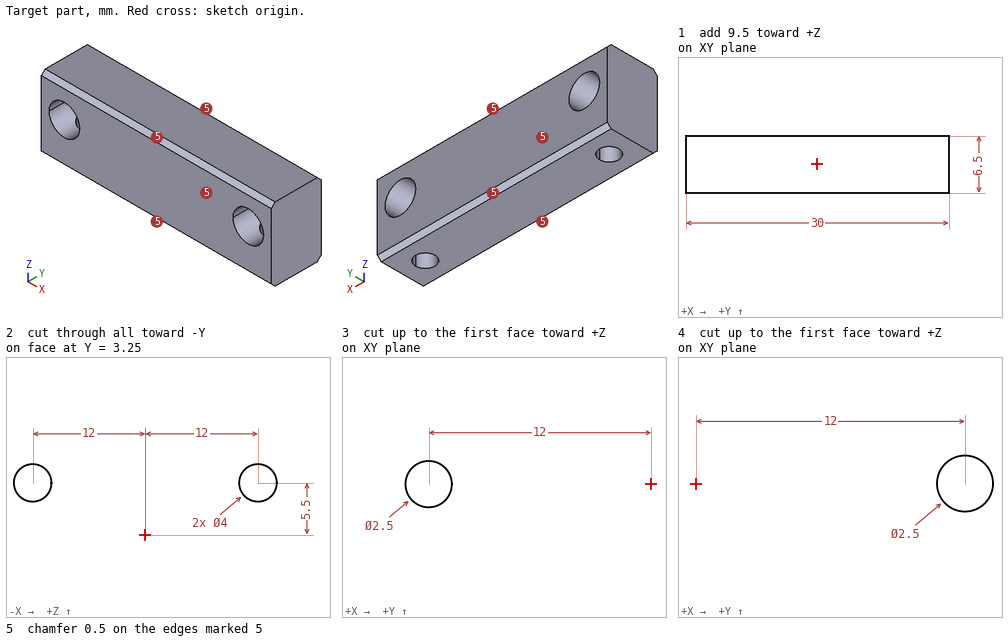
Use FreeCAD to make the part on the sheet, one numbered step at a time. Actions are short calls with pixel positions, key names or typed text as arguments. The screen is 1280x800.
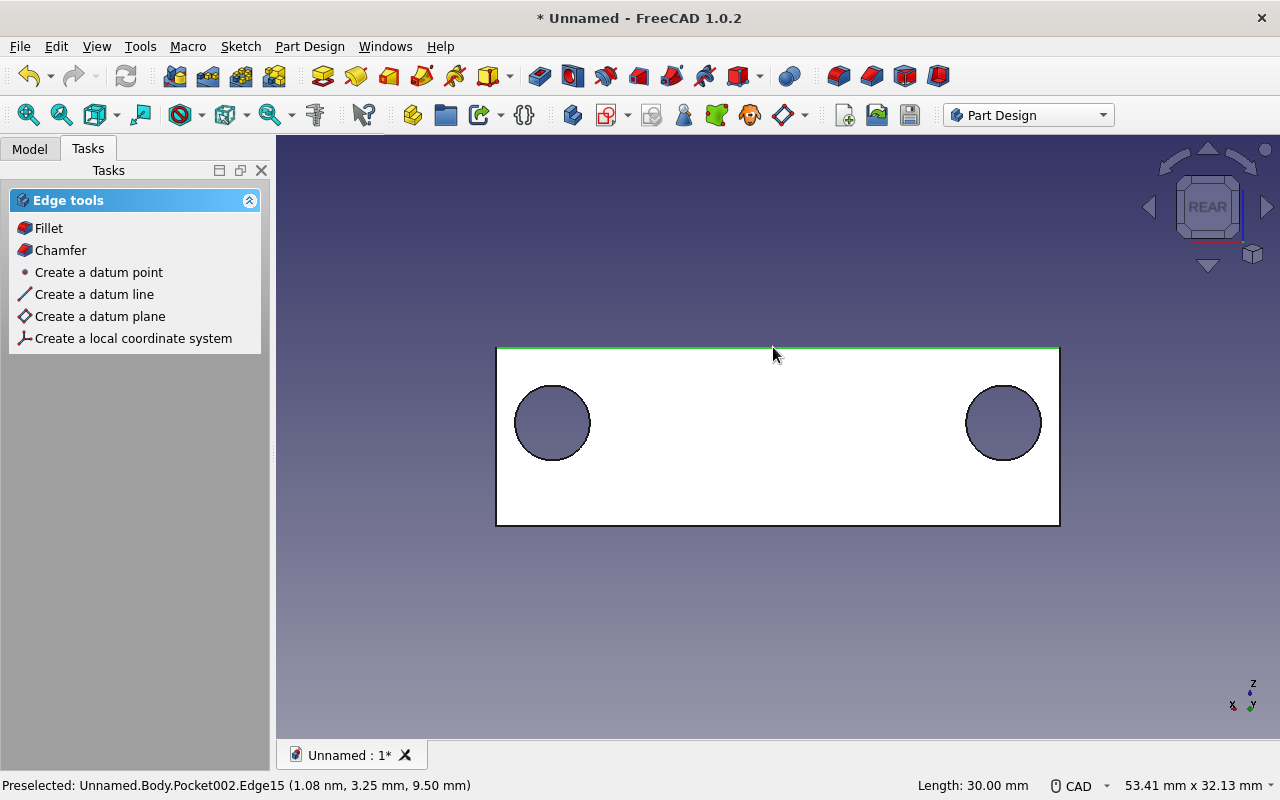
click(778, 525, ctrl)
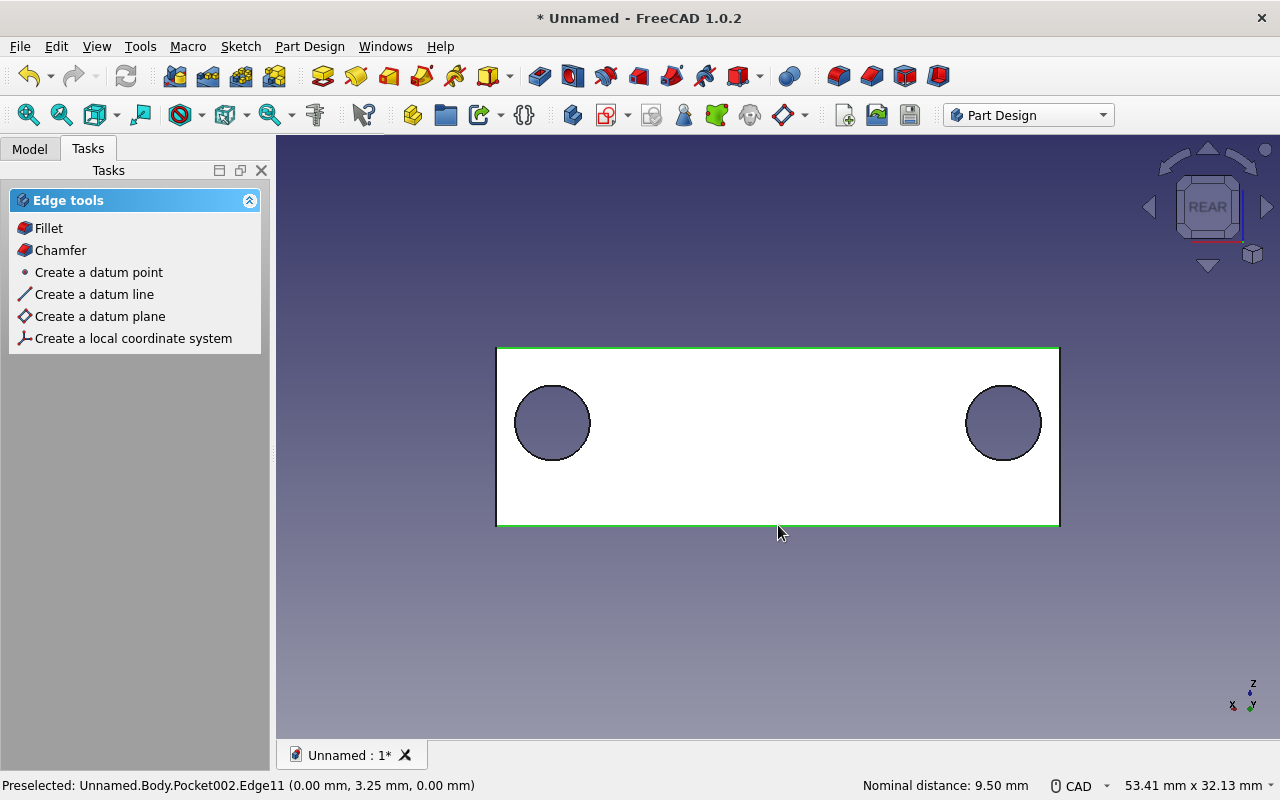
key(0)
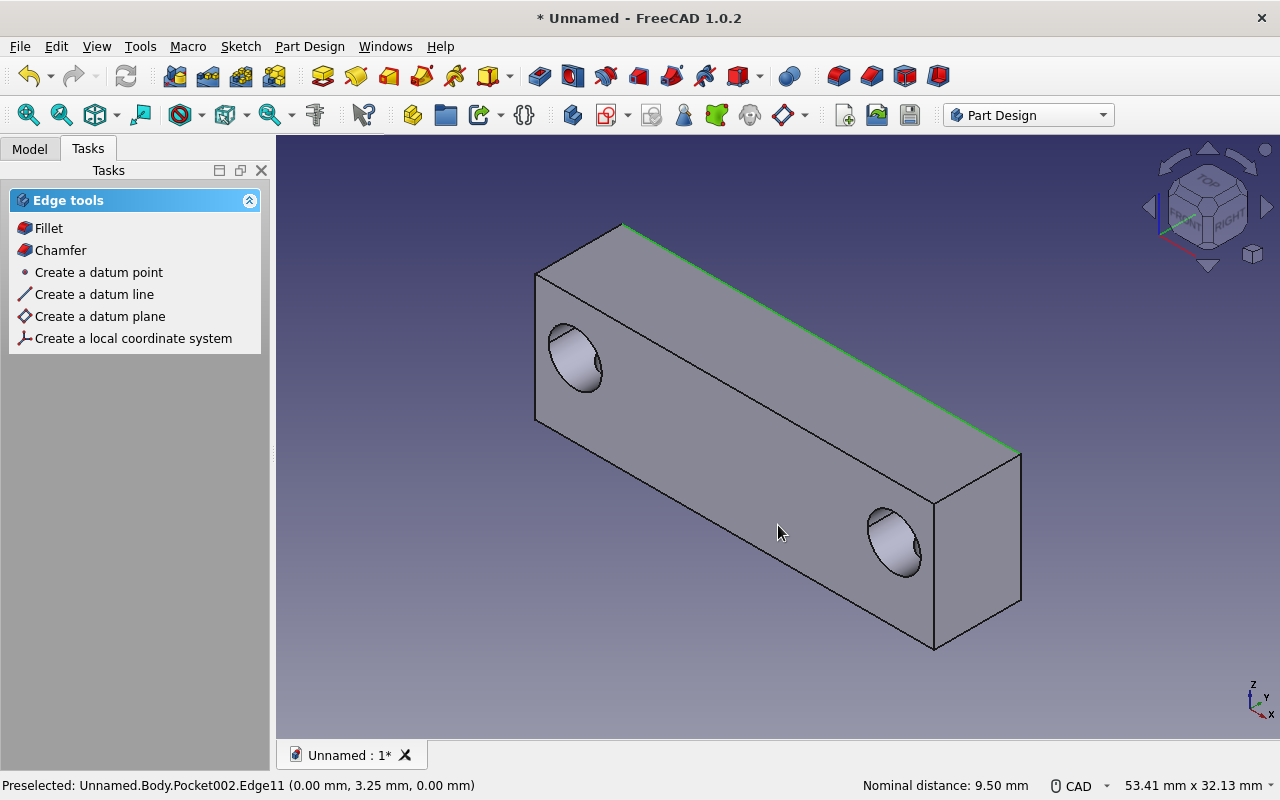
click(735, 388, ctrl)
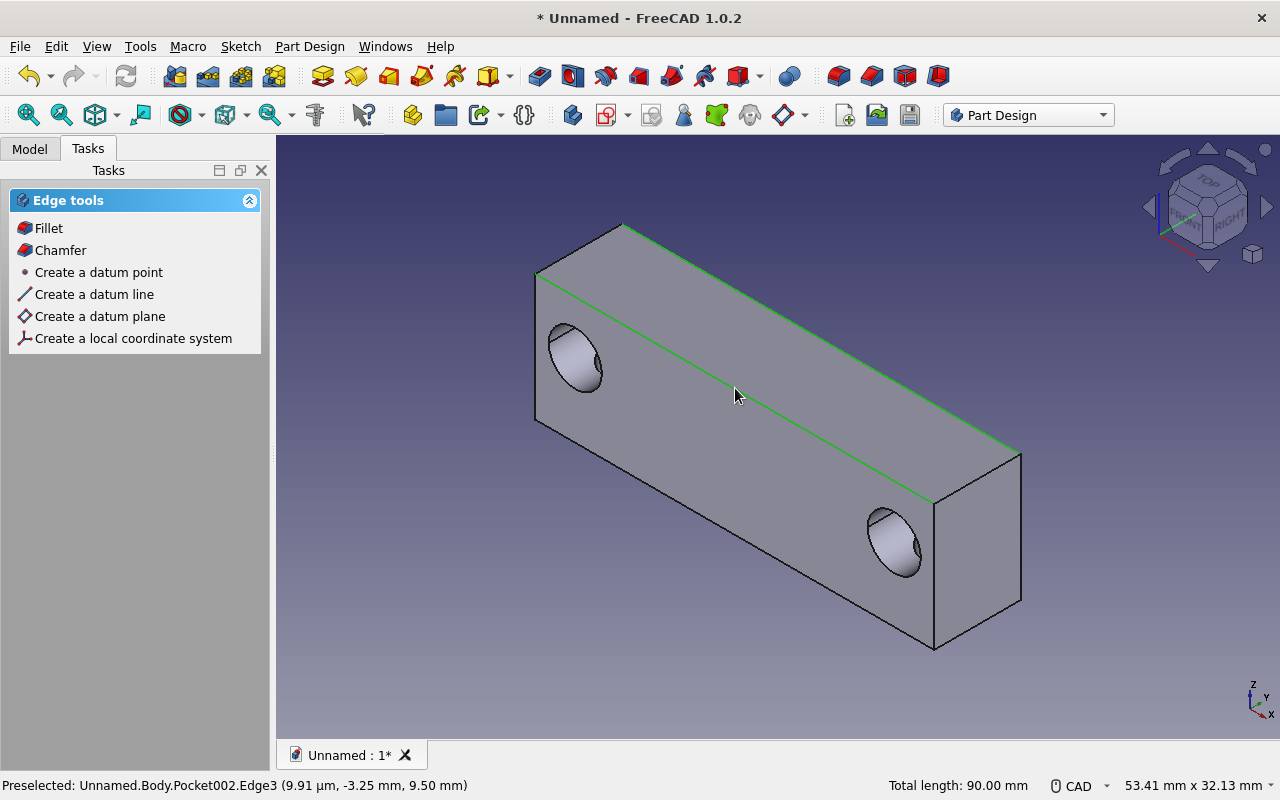
key(2)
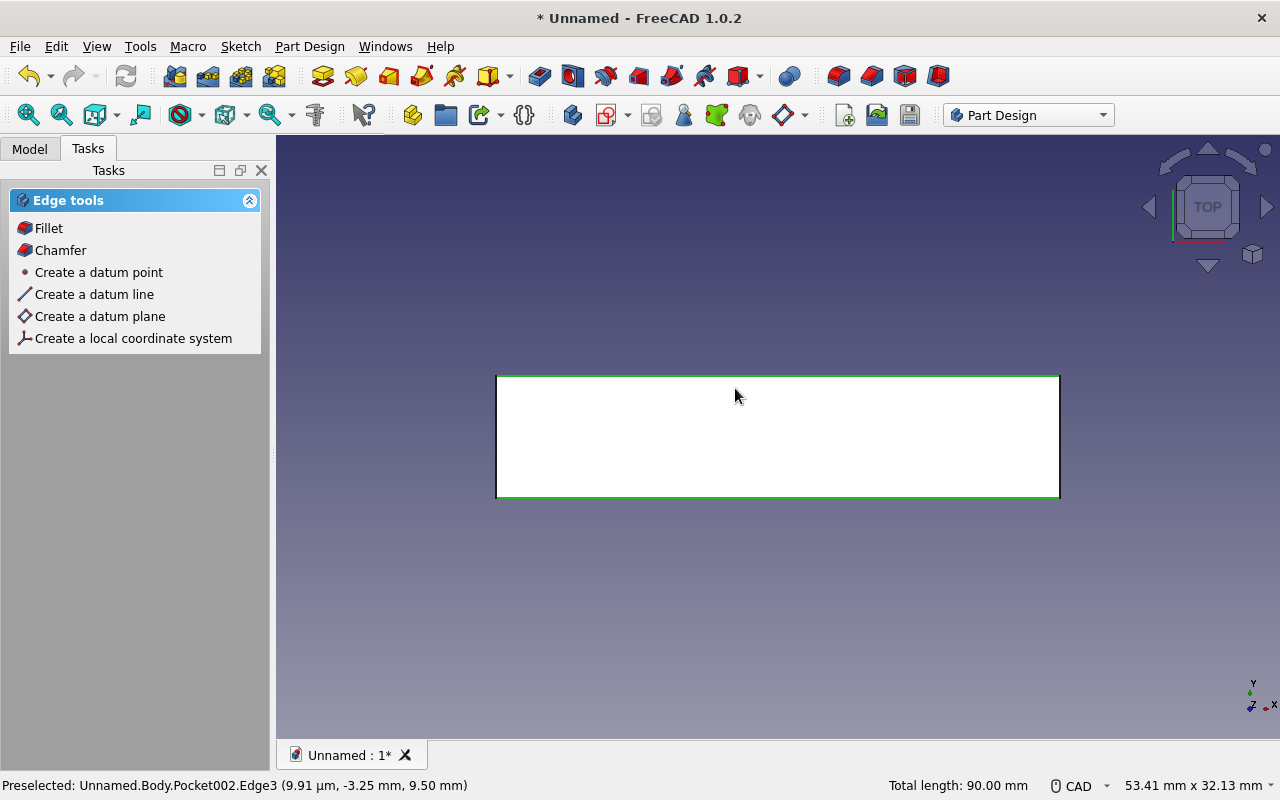
key(1)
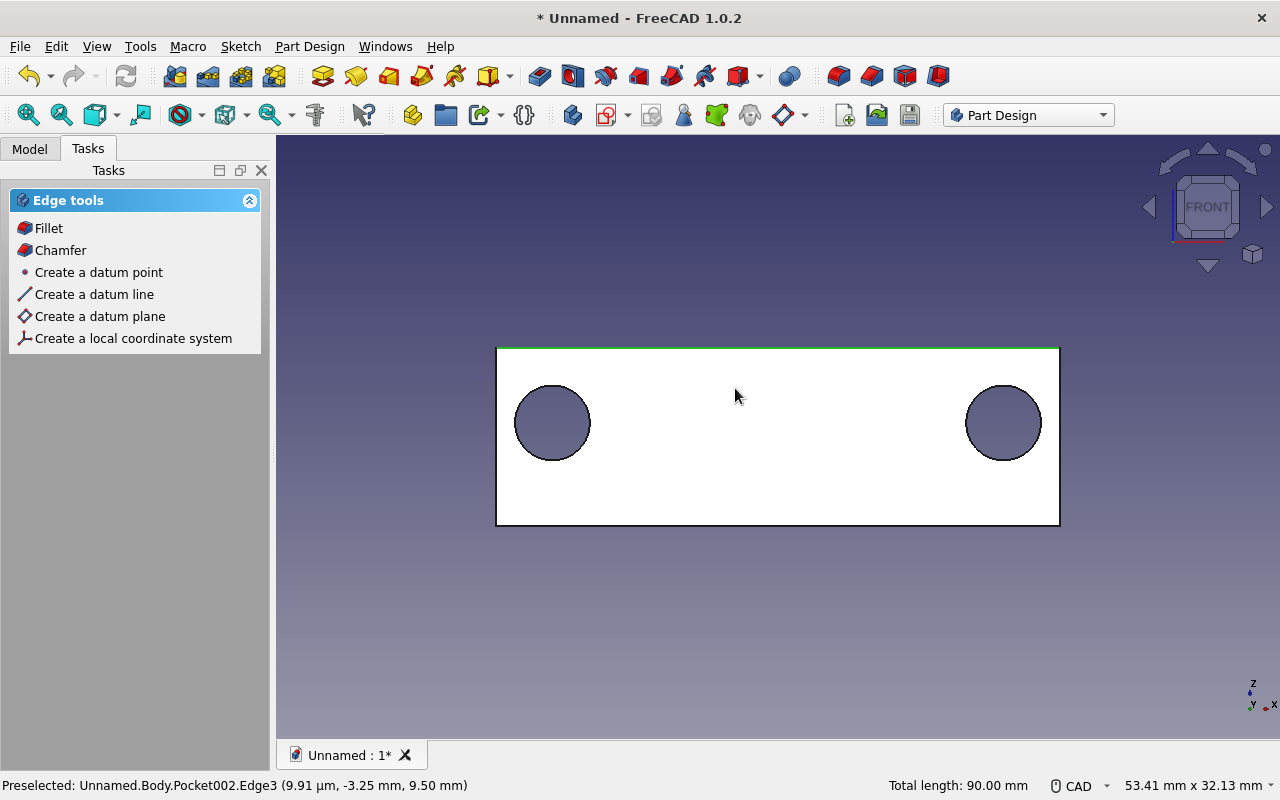
click(778, 525, ctrl)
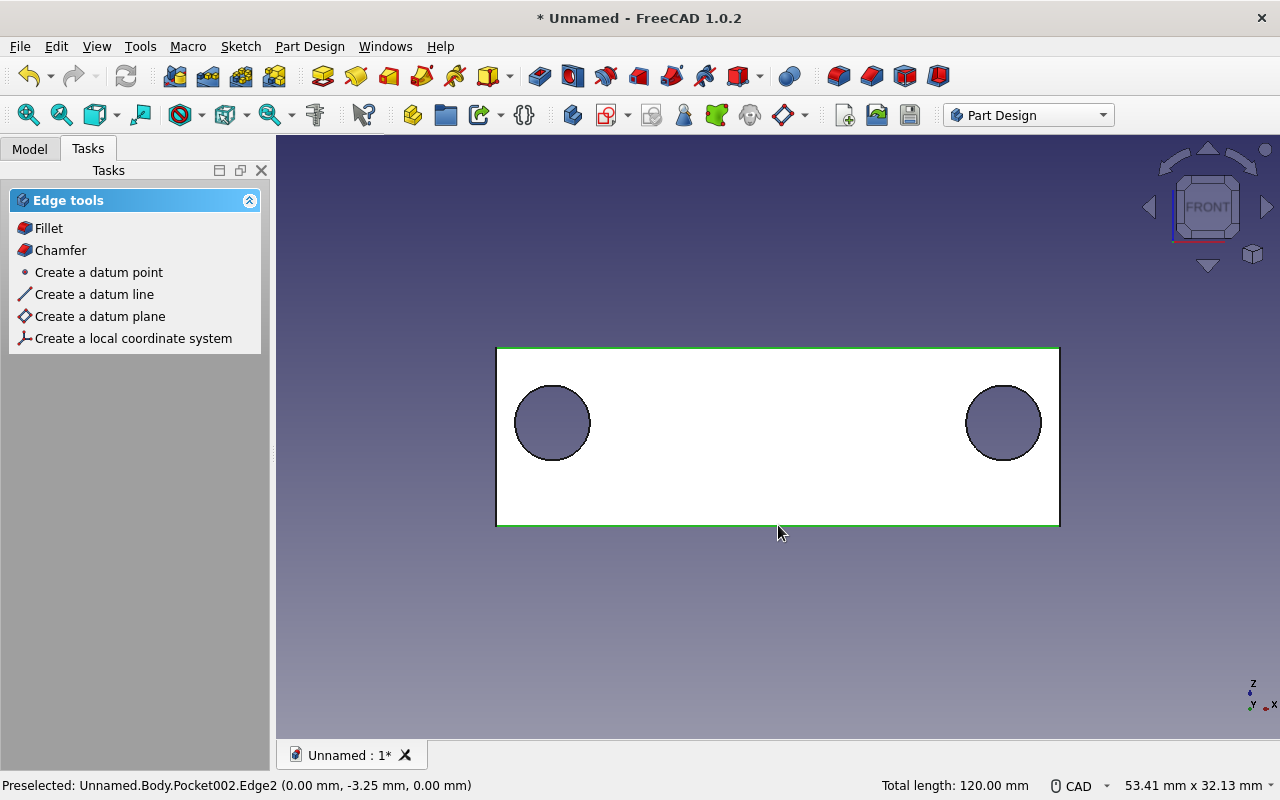
click(872, 76)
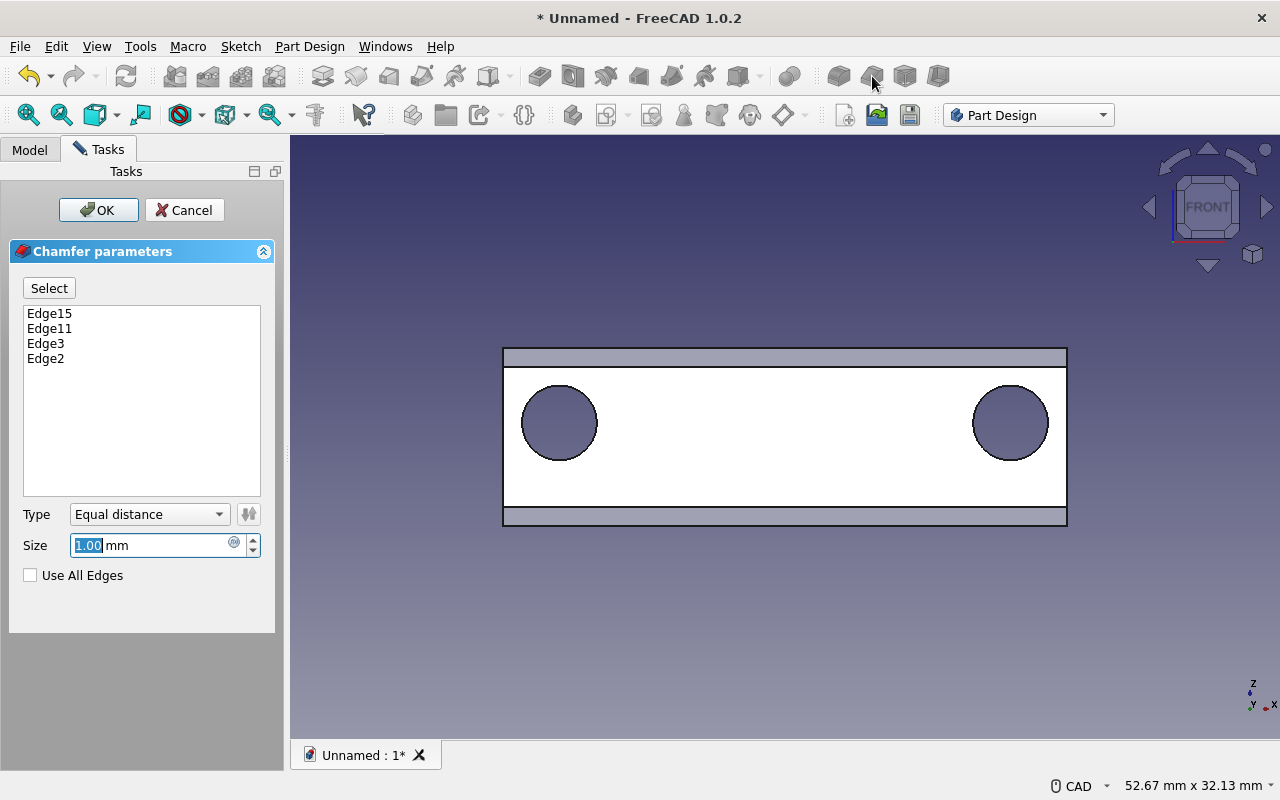
text(0.5)
key(Tab)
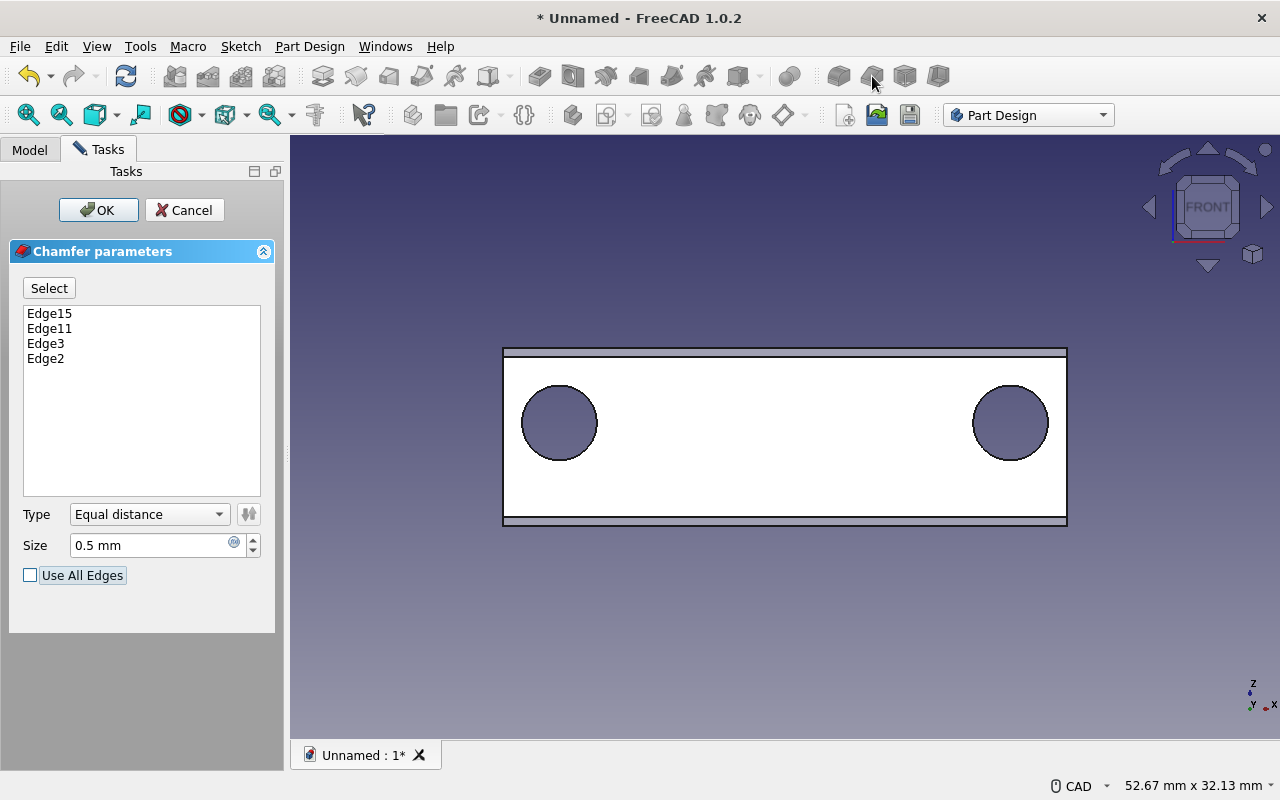
click(99, 210)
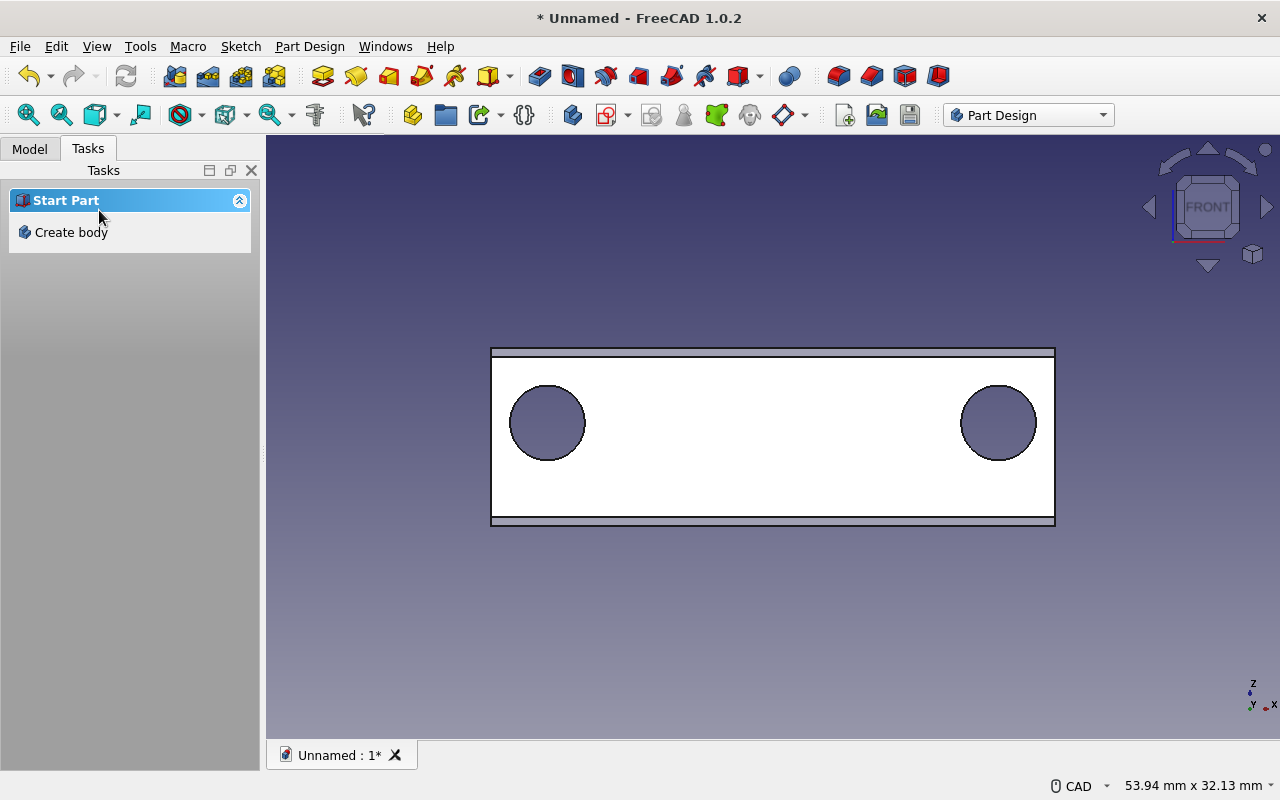
key(0)